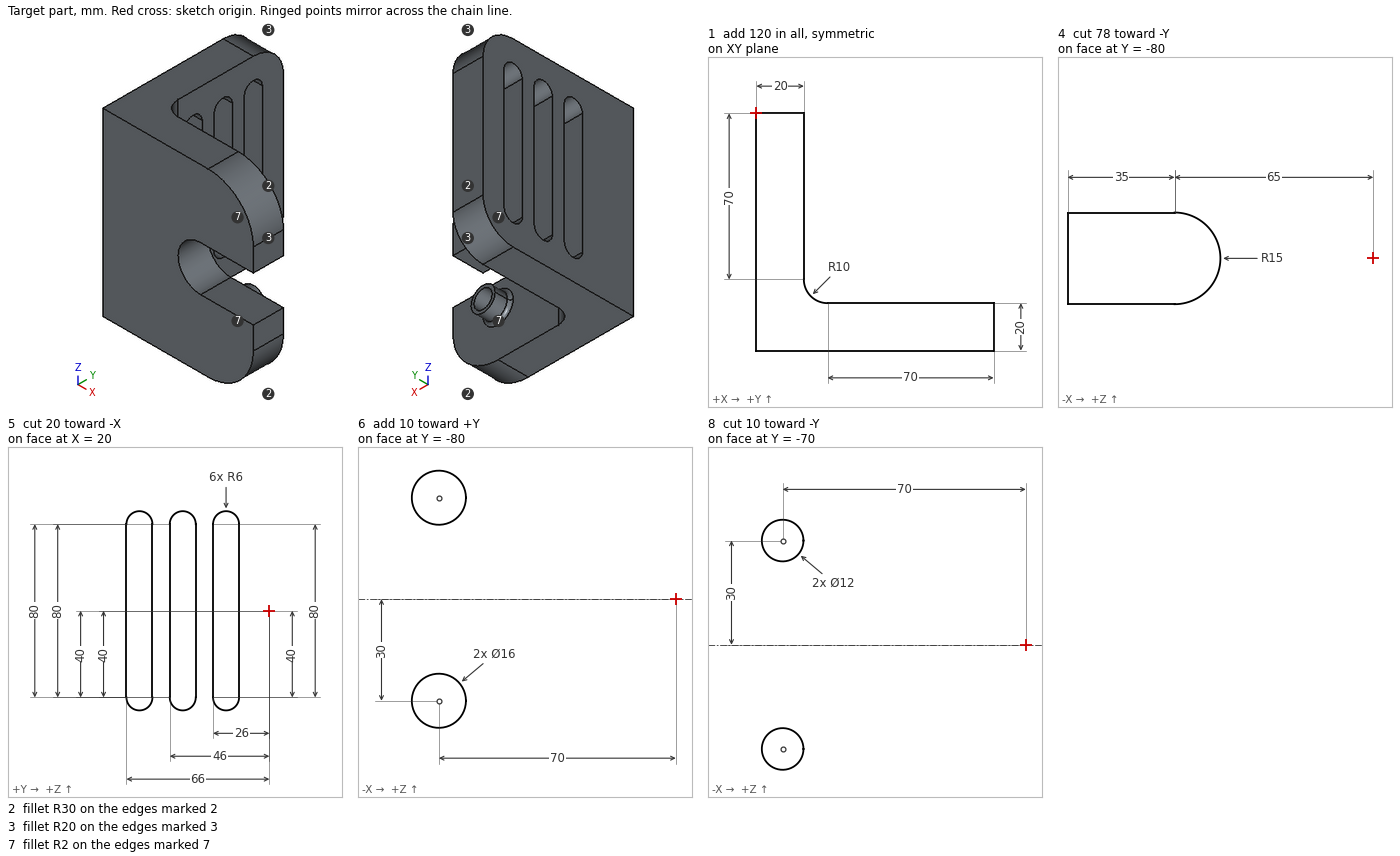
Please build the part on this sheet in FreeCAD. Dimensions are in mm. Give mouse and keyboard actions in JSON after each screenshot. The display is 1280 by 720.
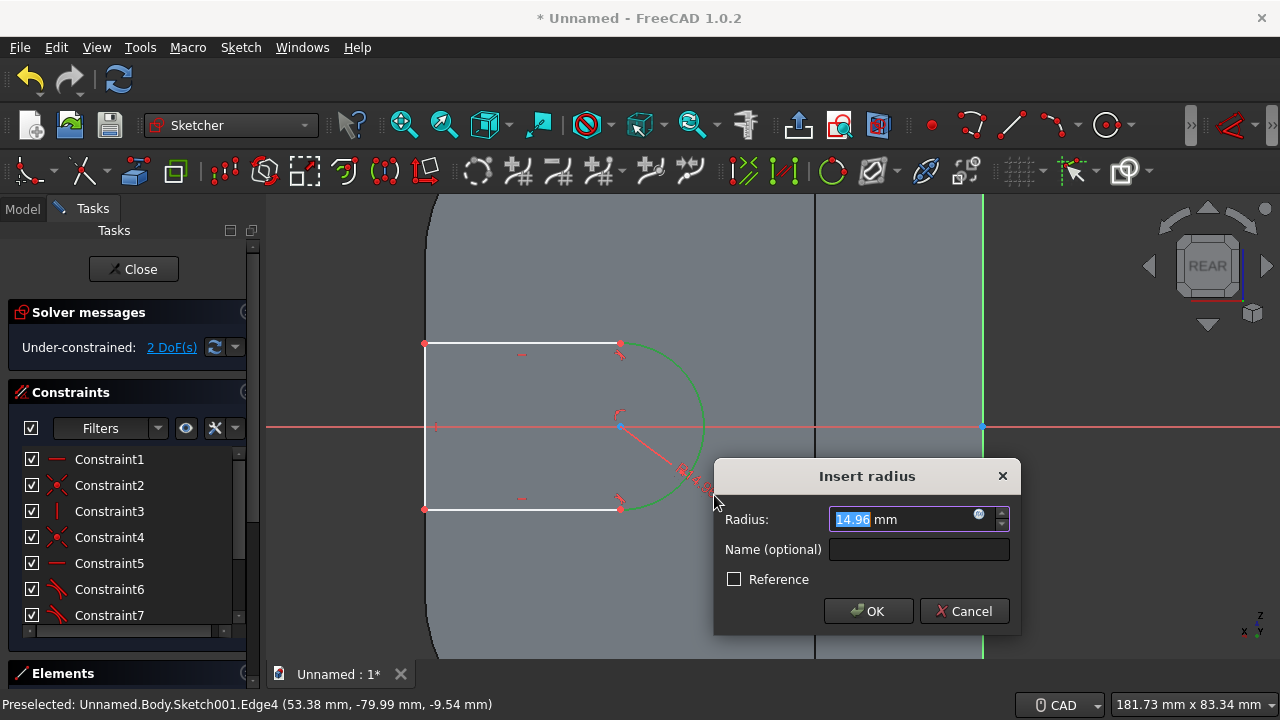
{"action": "type", "text": "15"}
{"action": "key", "text": "Return"}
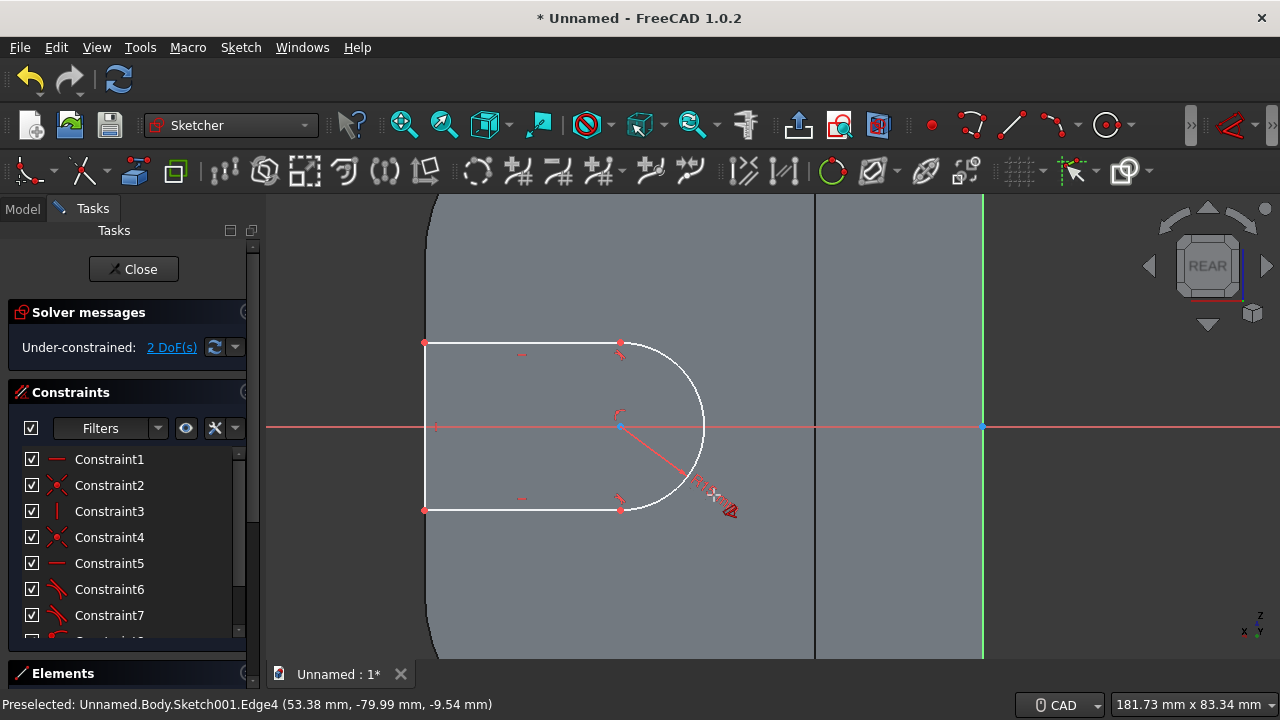
{"action": "left_click", "coordinate": [562, 343]}
{"action": "left_click", "coordinate": [523, 309]}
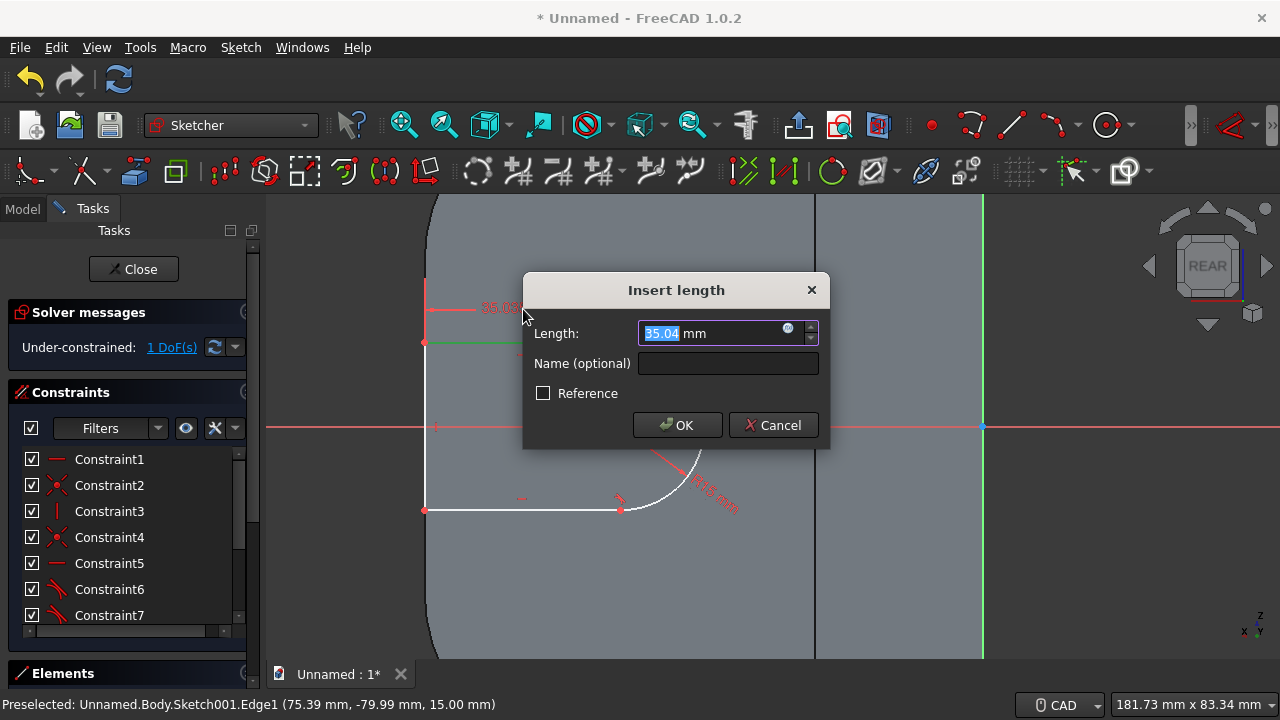
{"action": "type", "text": "35"}
{"action": "key", "text": "Return"}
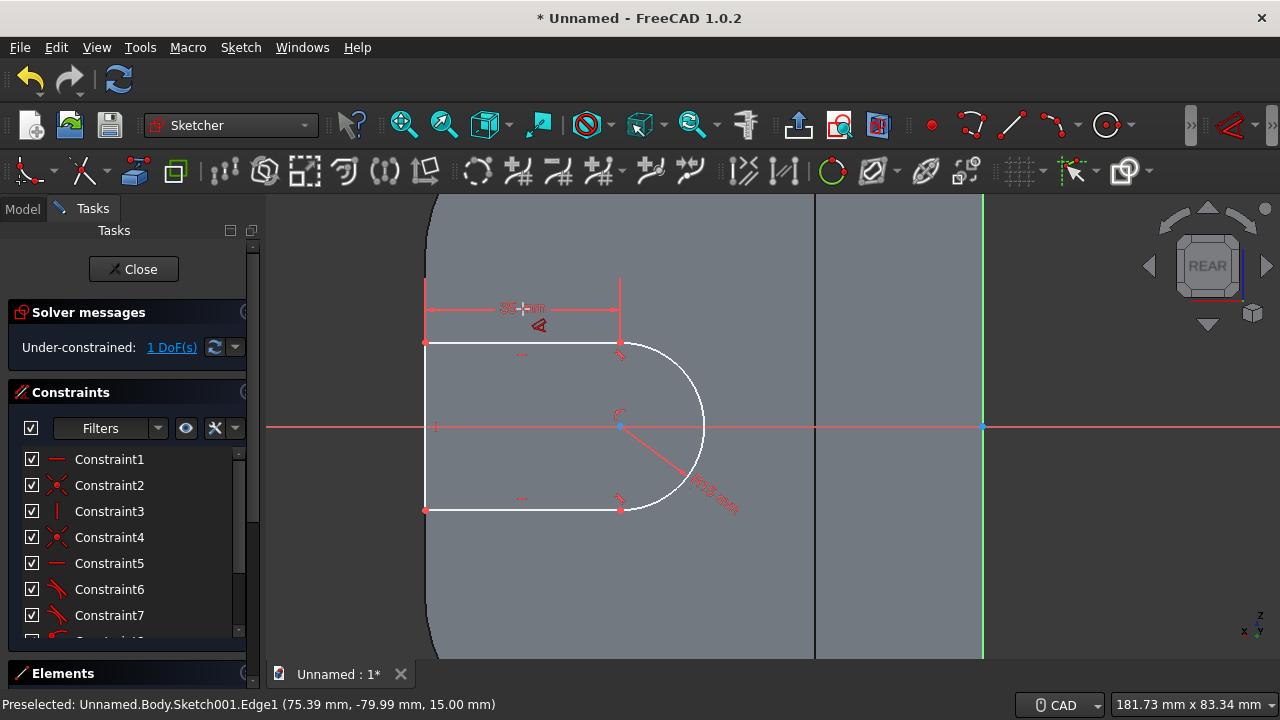
{"action": "left_click", "coordinate": [620, 343]}
{"action": "left_click", "coordinate": [802, 309]}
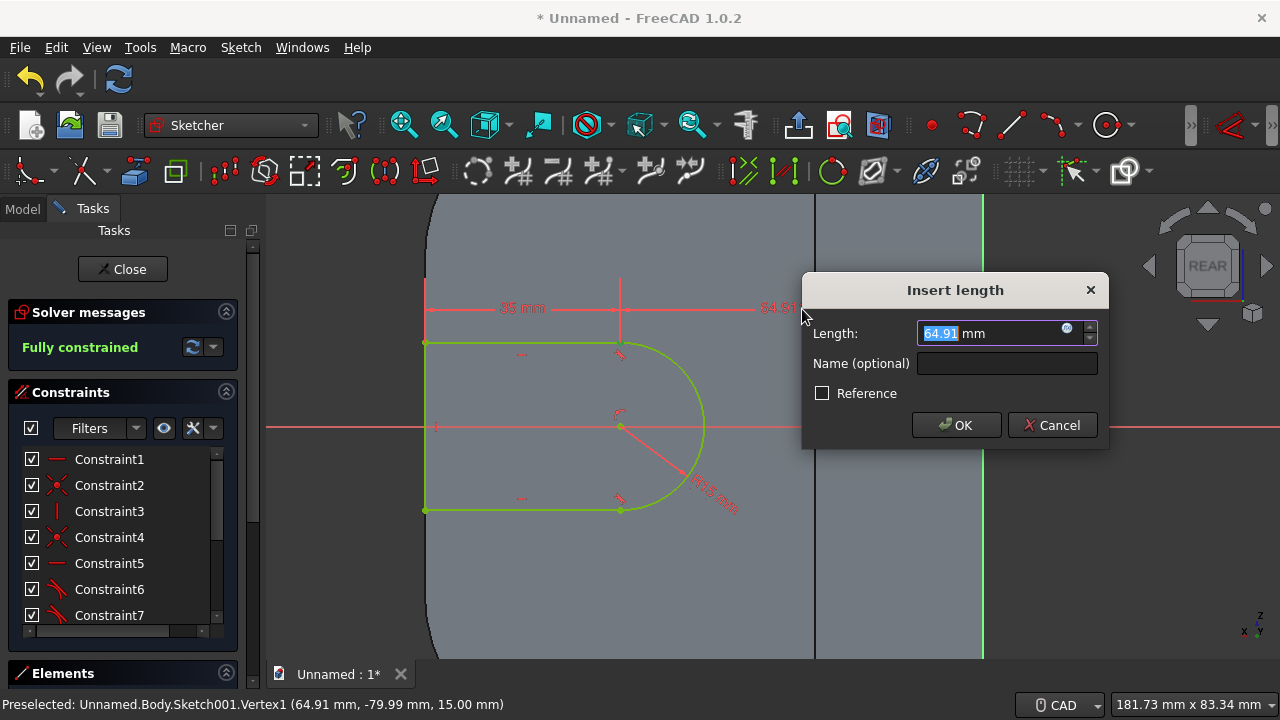
{"action": "type", "text": "65"}
{"action": "key", "text": "Return"}
{"action": "key", "text": "Escape"}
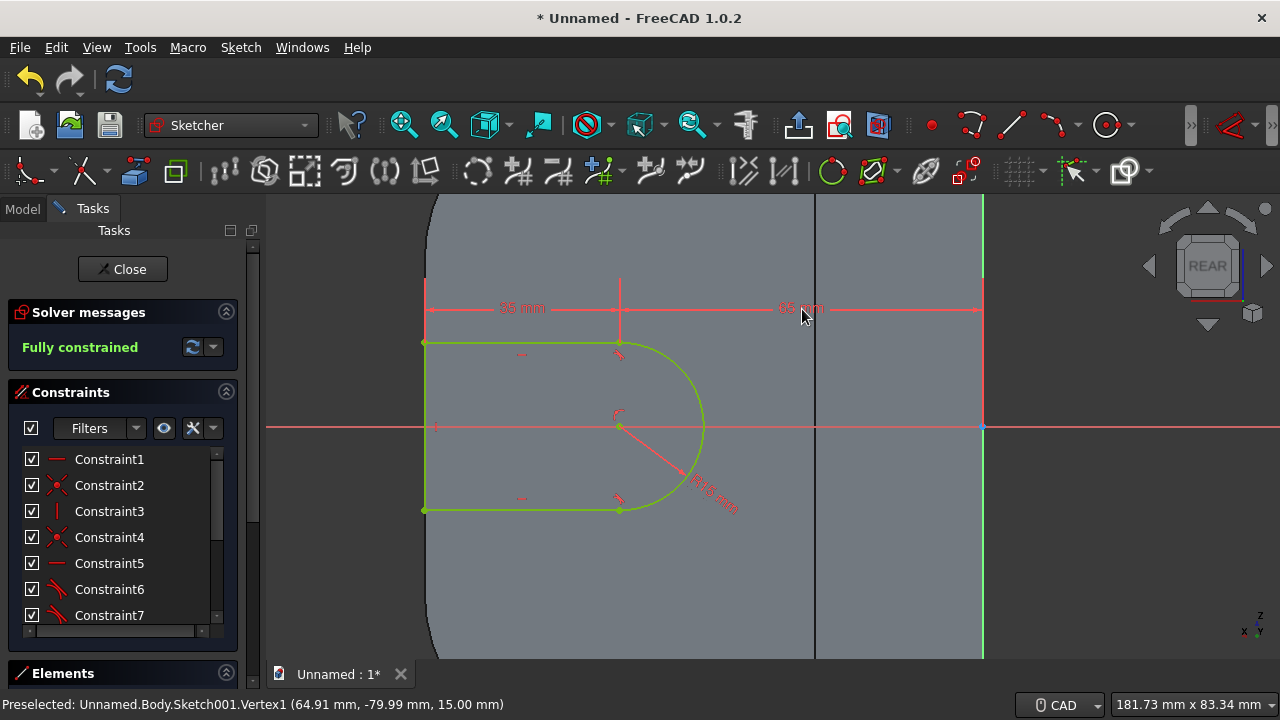
{"action": "left_click", "coordinate": [123, 269]}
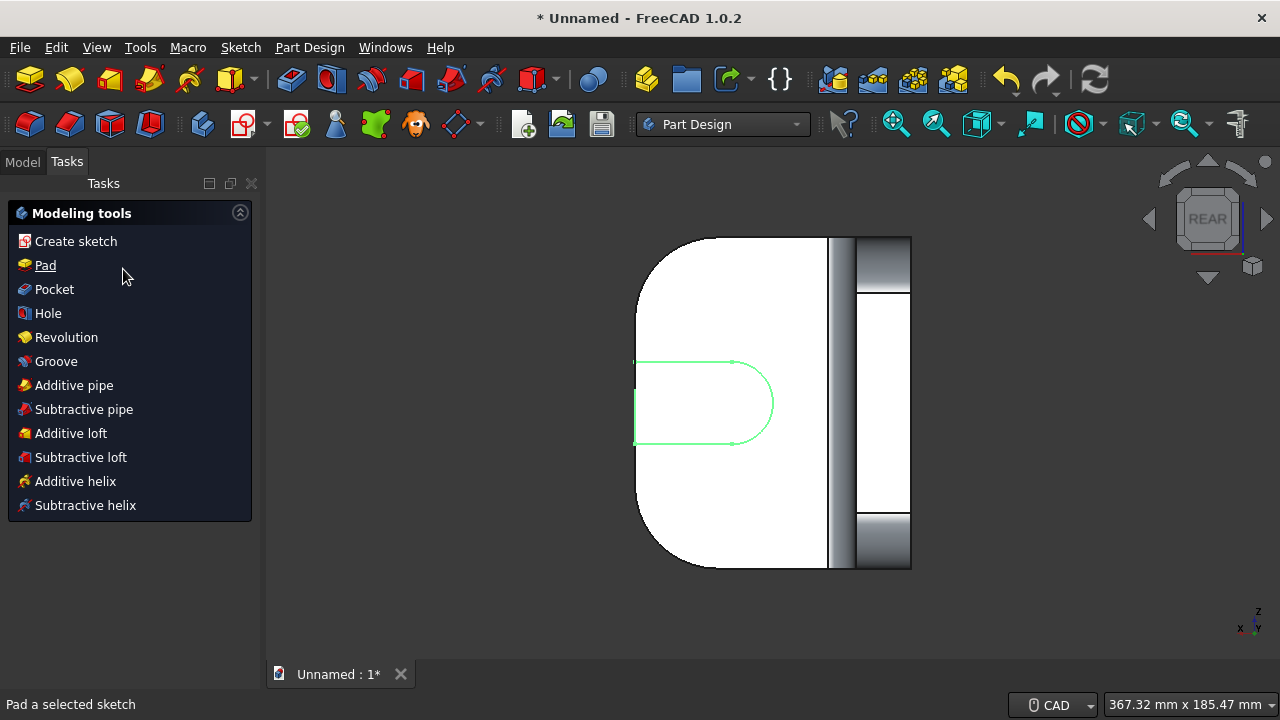
{"action": "left_click", "coordinate": [292, 80]}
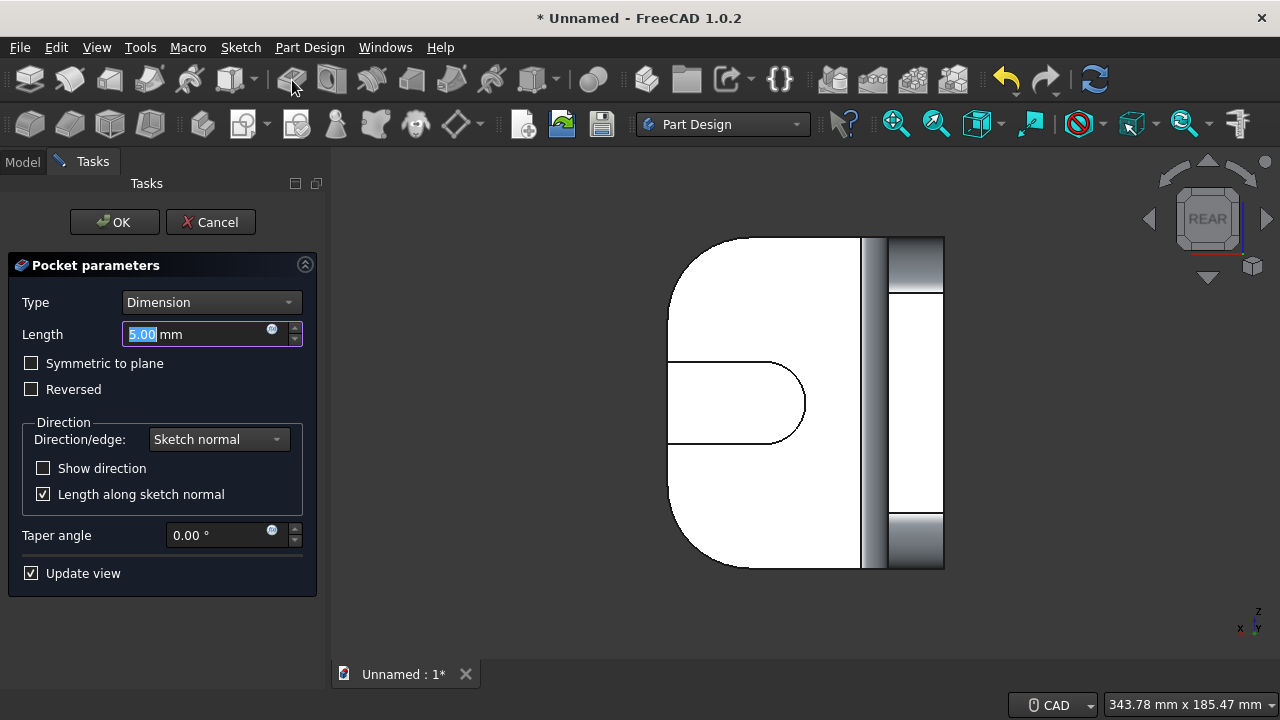
{"action": "type", "text": "78"}
{"action": "key", "text": "Tab"}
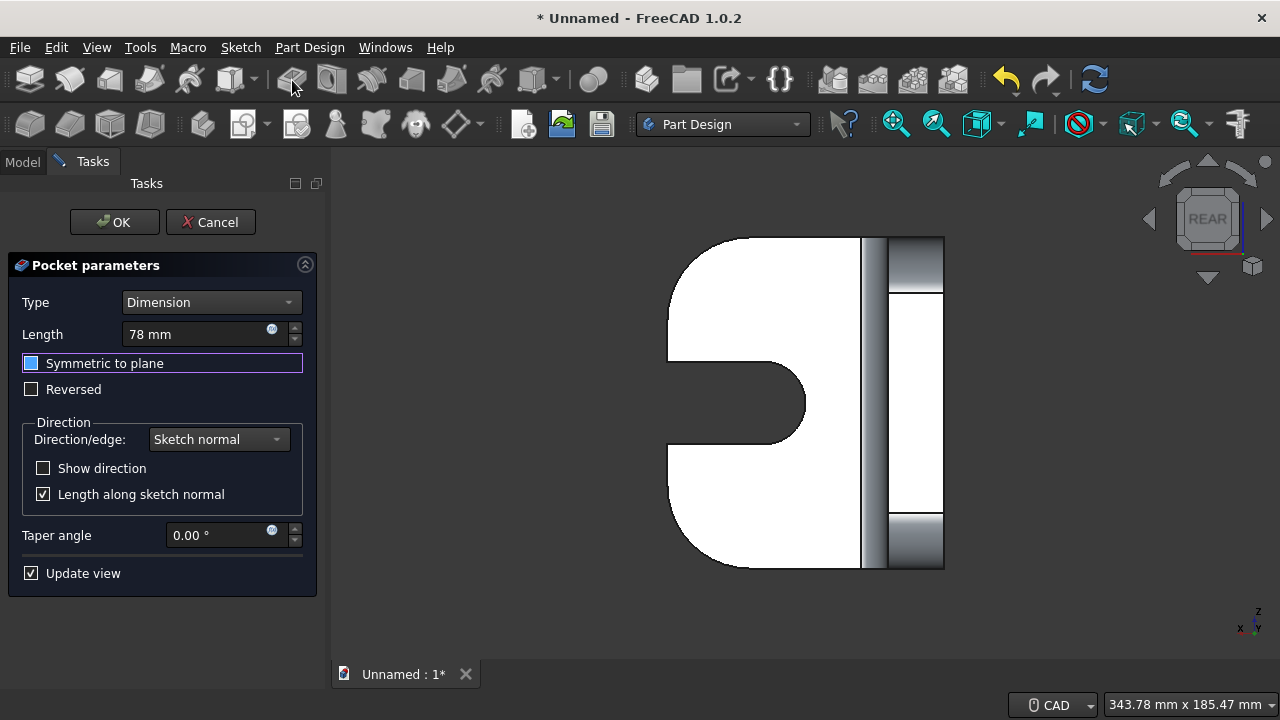
{"action": "left_click", "coordinate": [115, 222]}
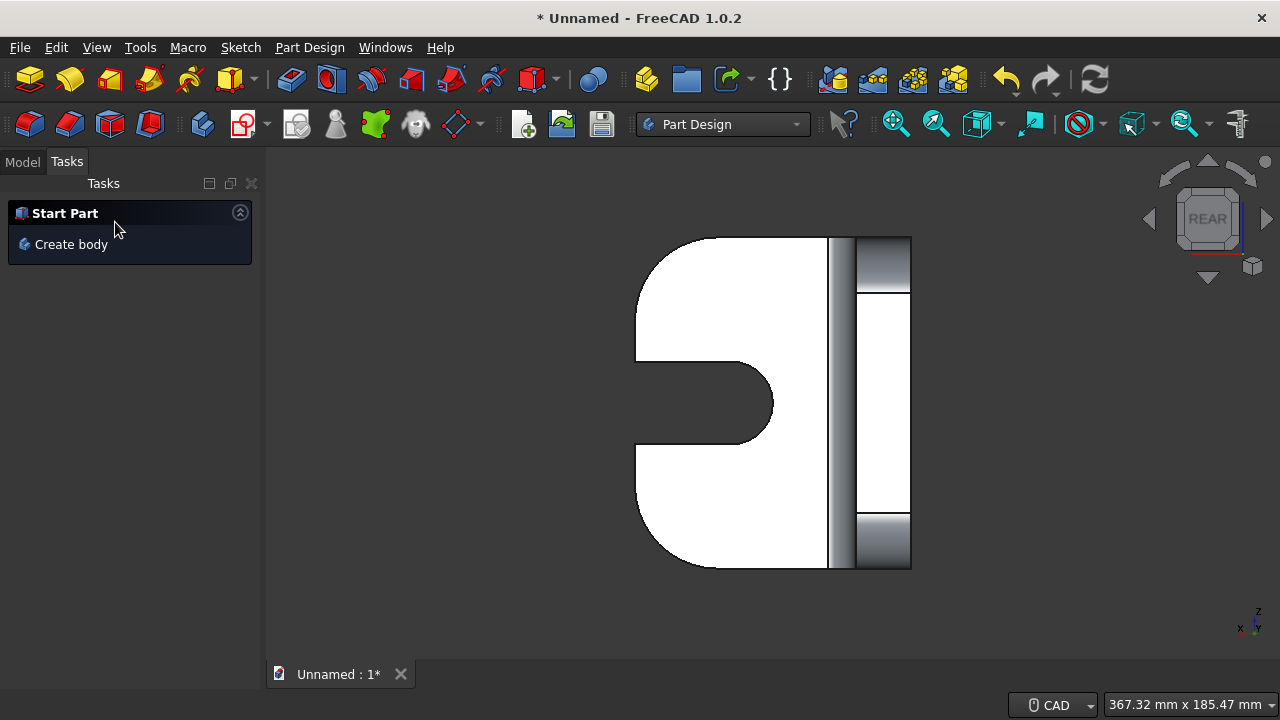
{"action": "key", "text": "0"}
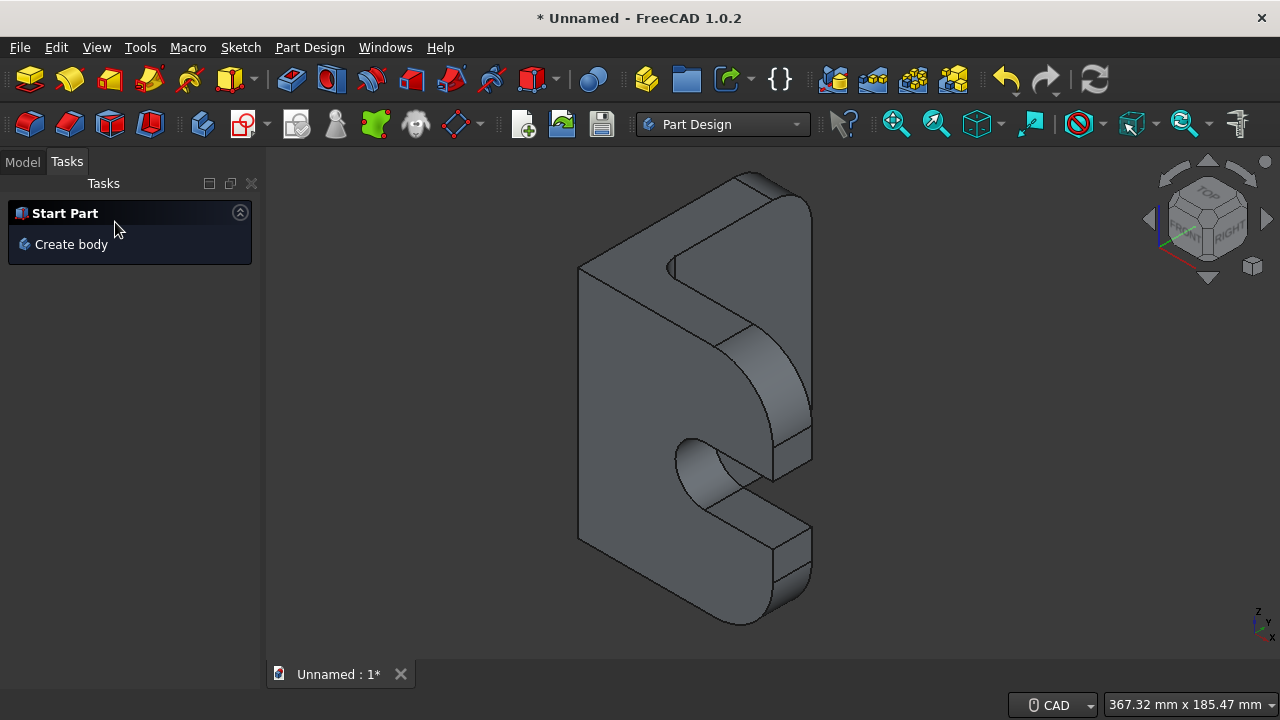
{"action": "left_click", "coordinate": [744, 274]}